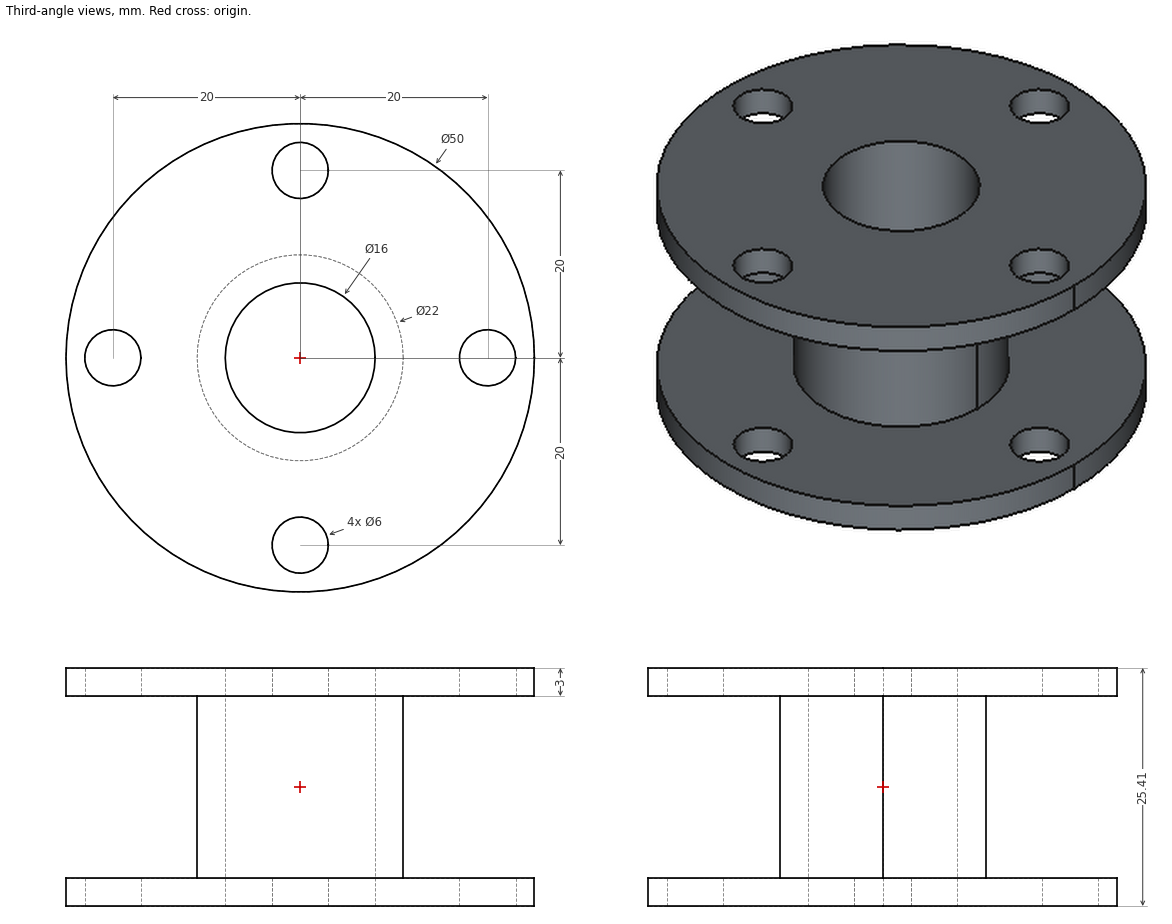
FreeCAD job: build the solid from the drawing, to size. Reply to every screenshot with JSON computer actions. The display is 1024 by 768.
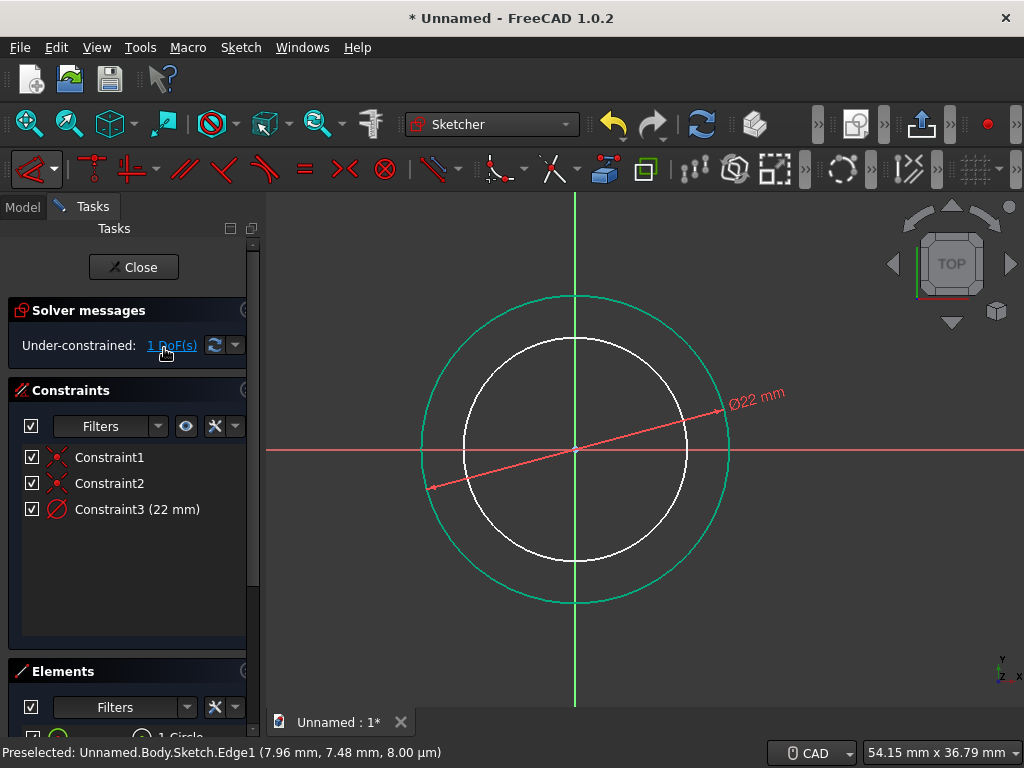
{"action": "left_click", "coordinate": [654, 370]}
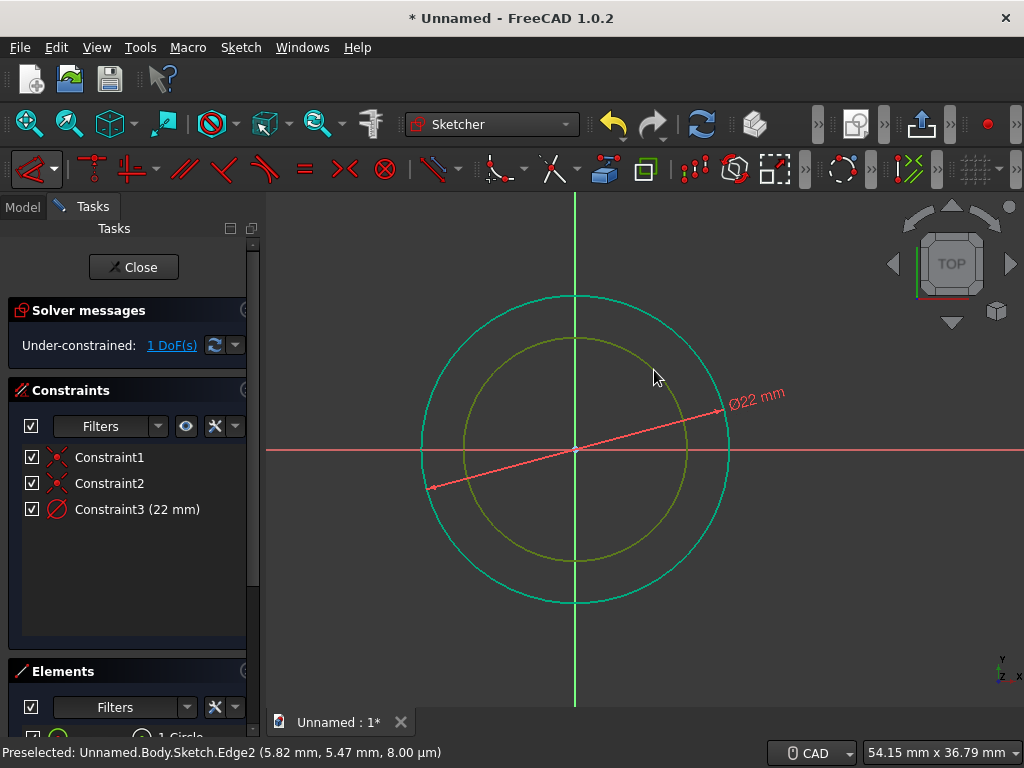
{"action": "left_click", "coordinate": [56, 170]}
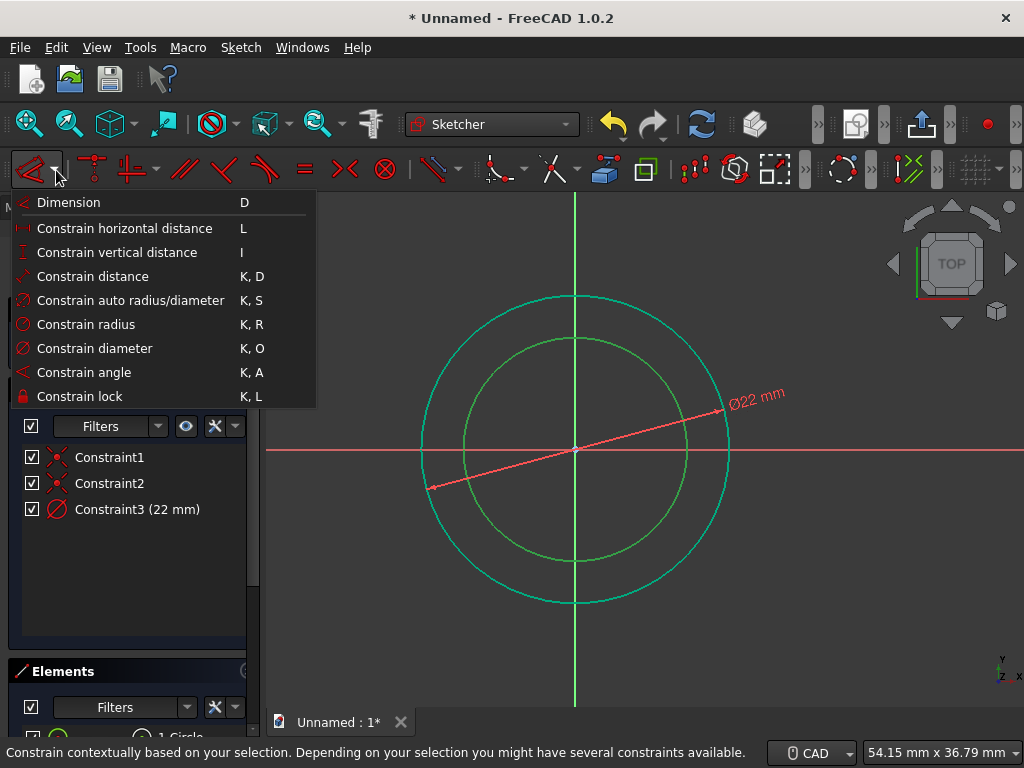
{"action": "left_click", "coordinate": [164, 348]}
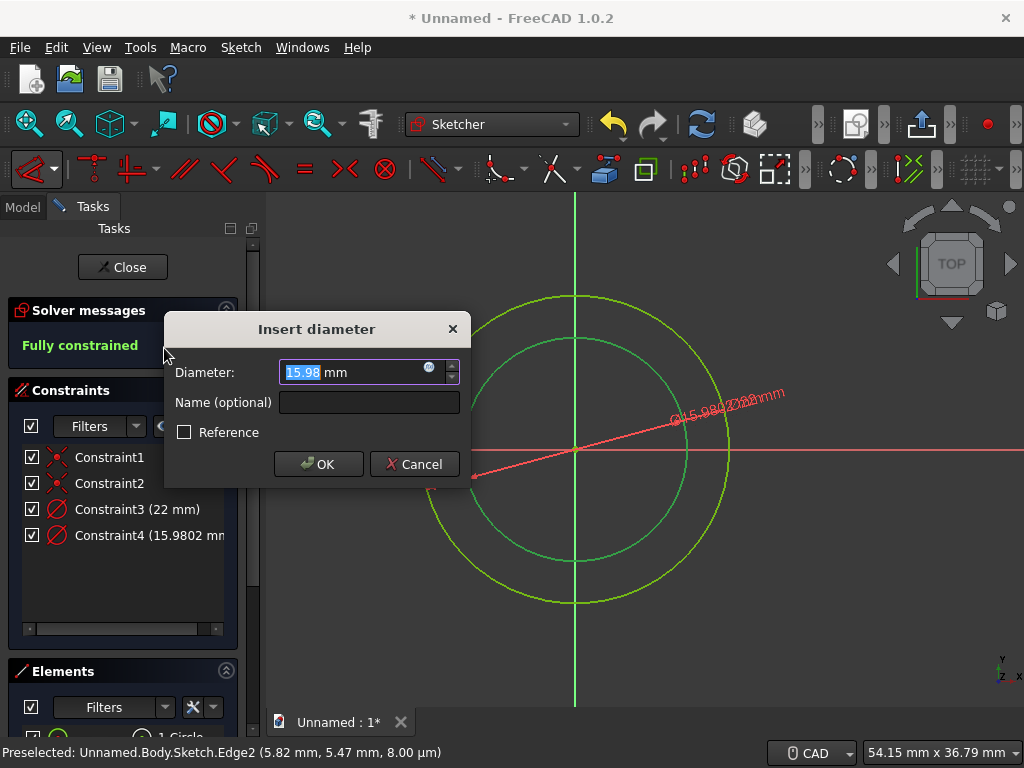
{"action": "type", "text": "16"}
{"action": "key", "text": "Return"}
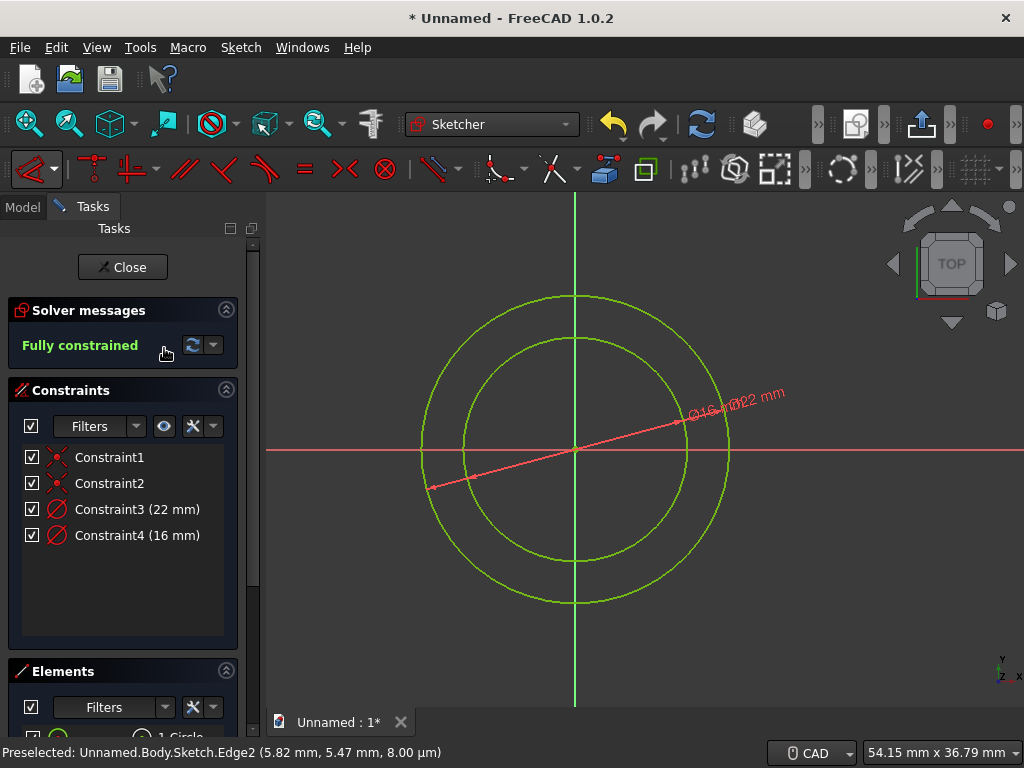
{"action": "left_click", "coordinate": [123, 267]}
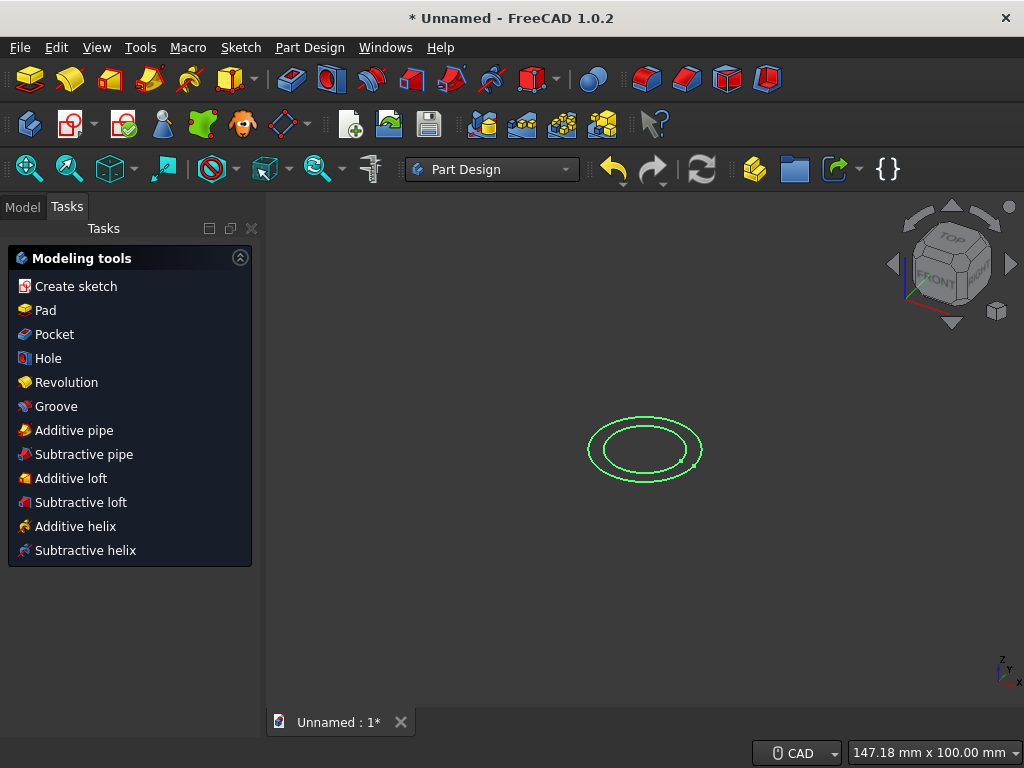
{"action": "left_click", "coordinate": [30, 80]}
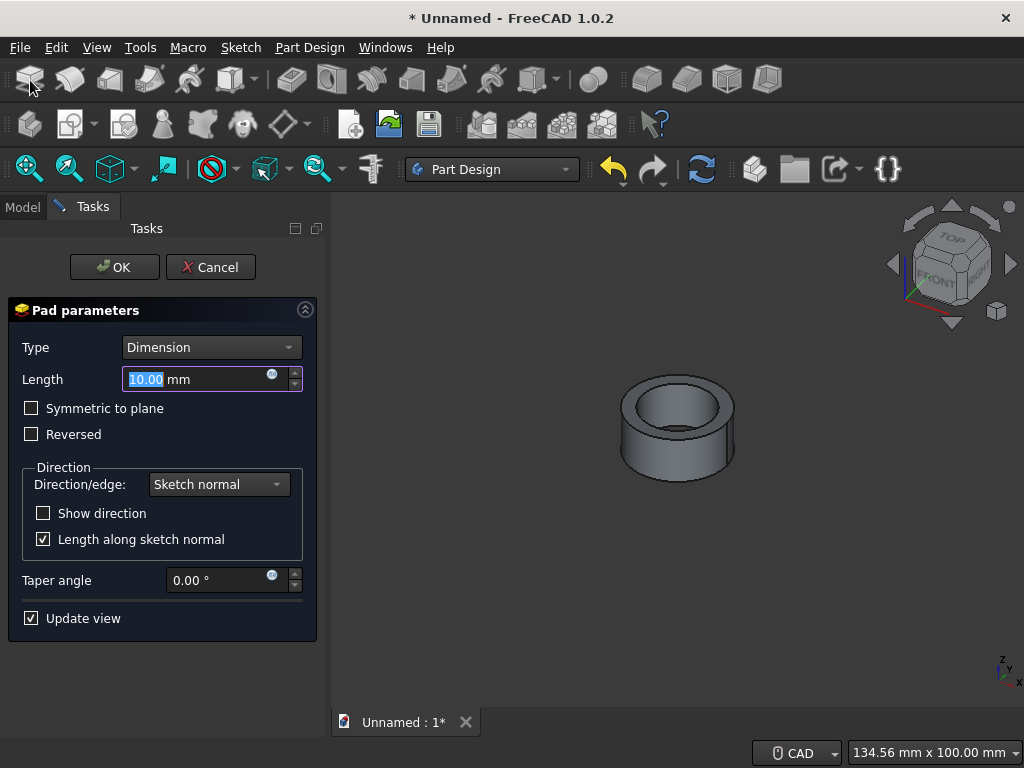
{"action": "type", "text": "25.41"}
{"action": "key", "text": "Tab"}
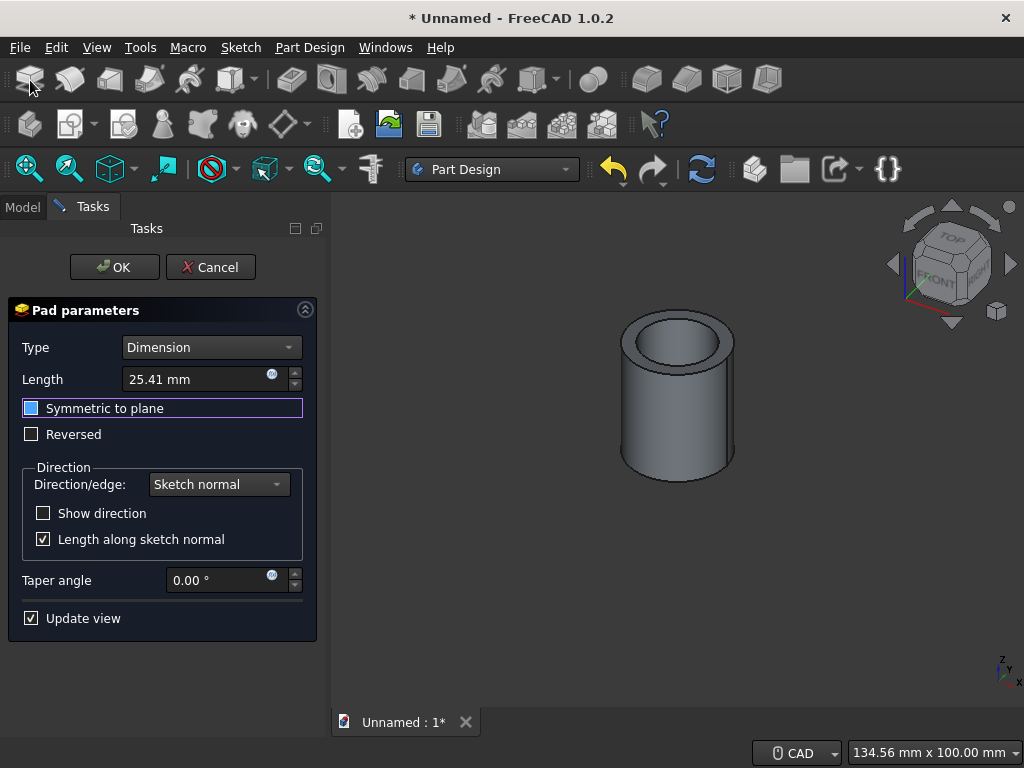
{"action": "left_click", "coordinate": [30, 408]}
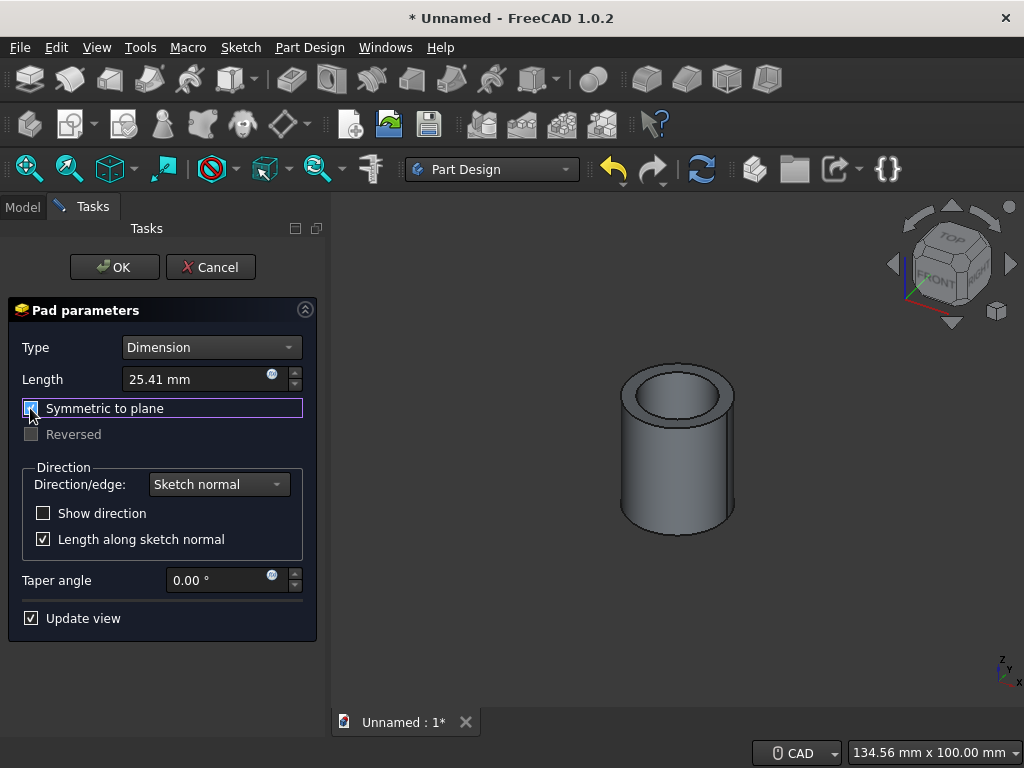
{"action": "left_click", "coordinate": [115, 267]}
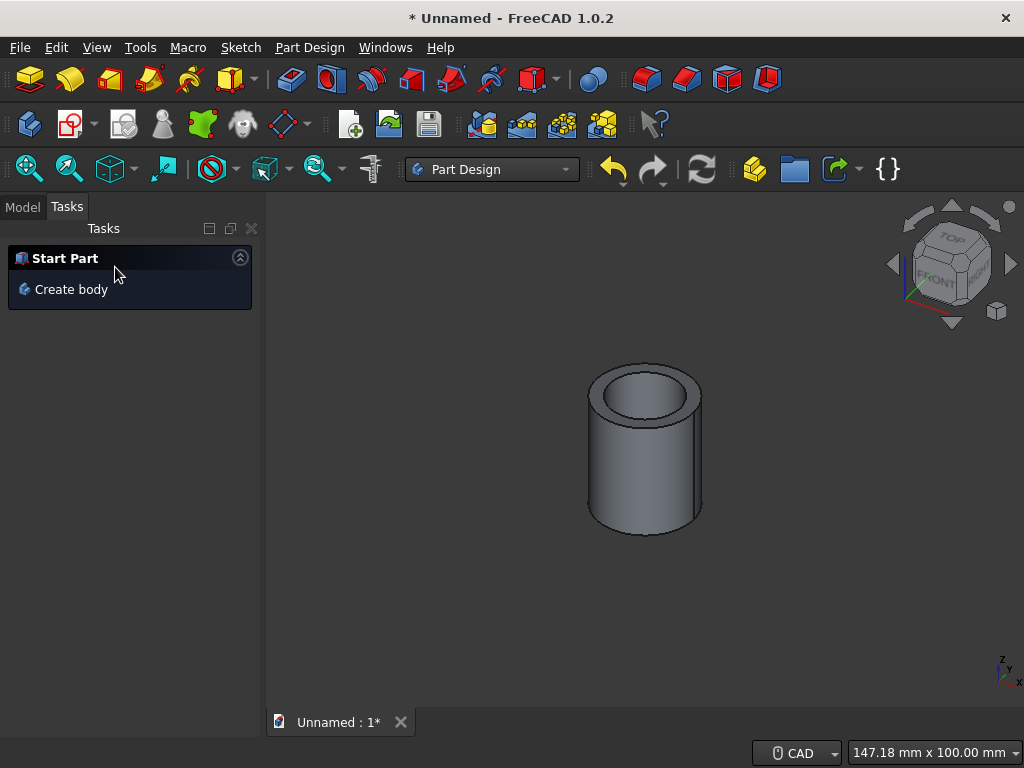
{"action": "left_click", "coordinate": [30, 170]}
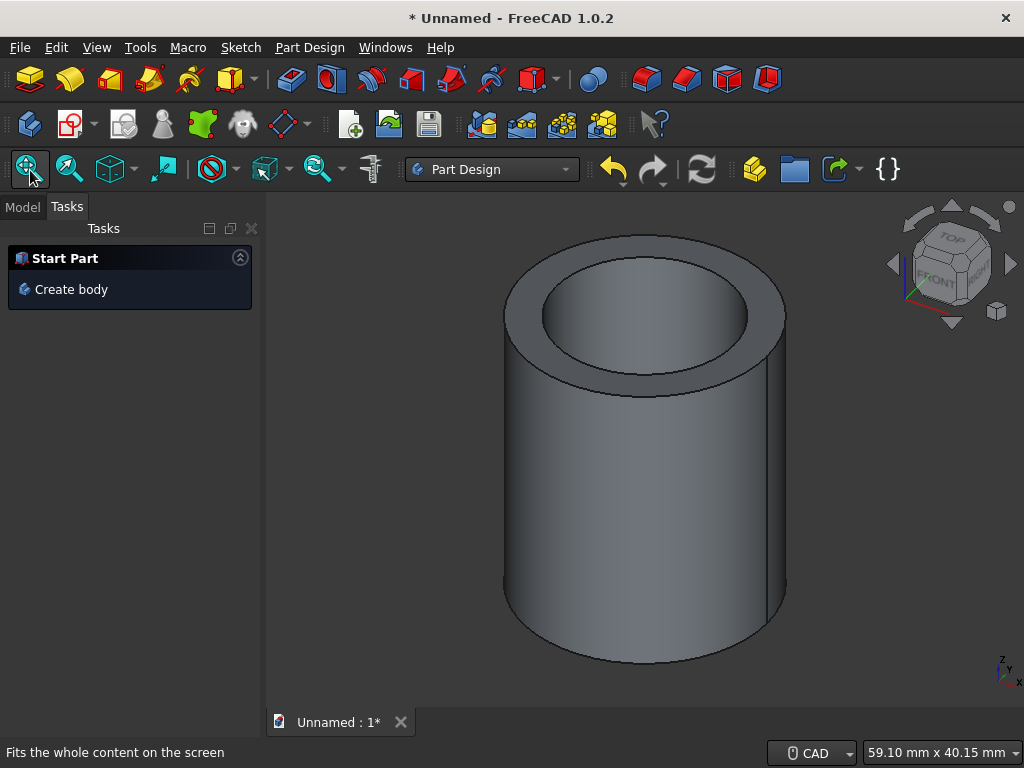
{"action": "left_click", "coordinate": [23, 206]}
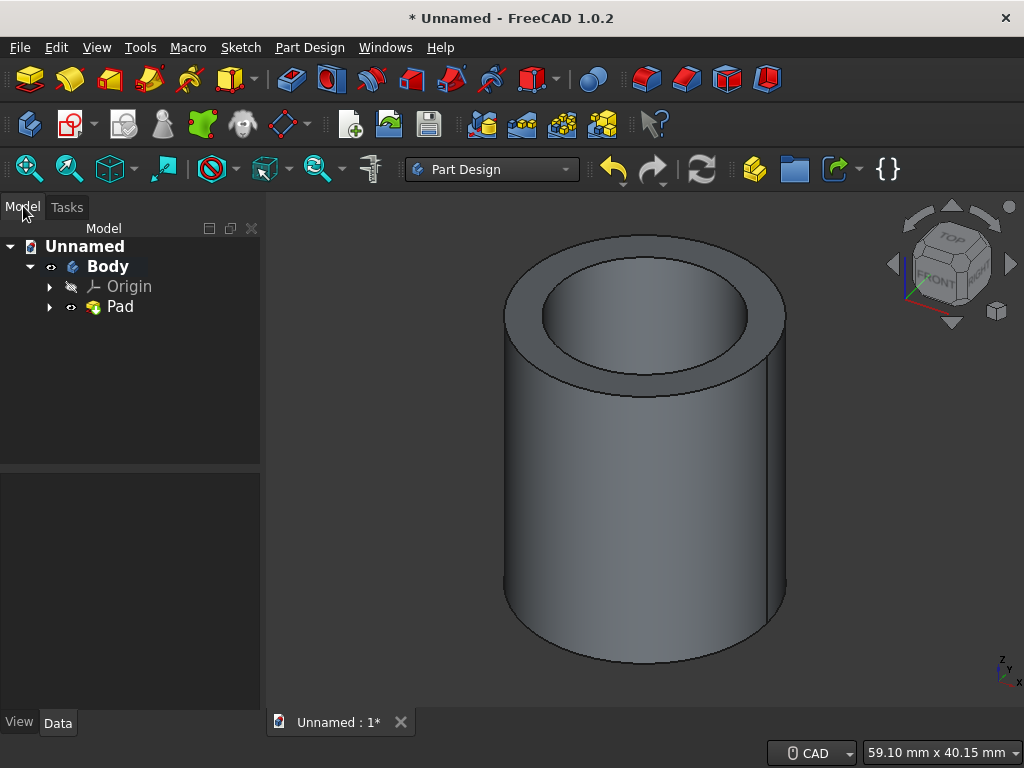
{"action": "left_click", "coordinate": [50, 287]}